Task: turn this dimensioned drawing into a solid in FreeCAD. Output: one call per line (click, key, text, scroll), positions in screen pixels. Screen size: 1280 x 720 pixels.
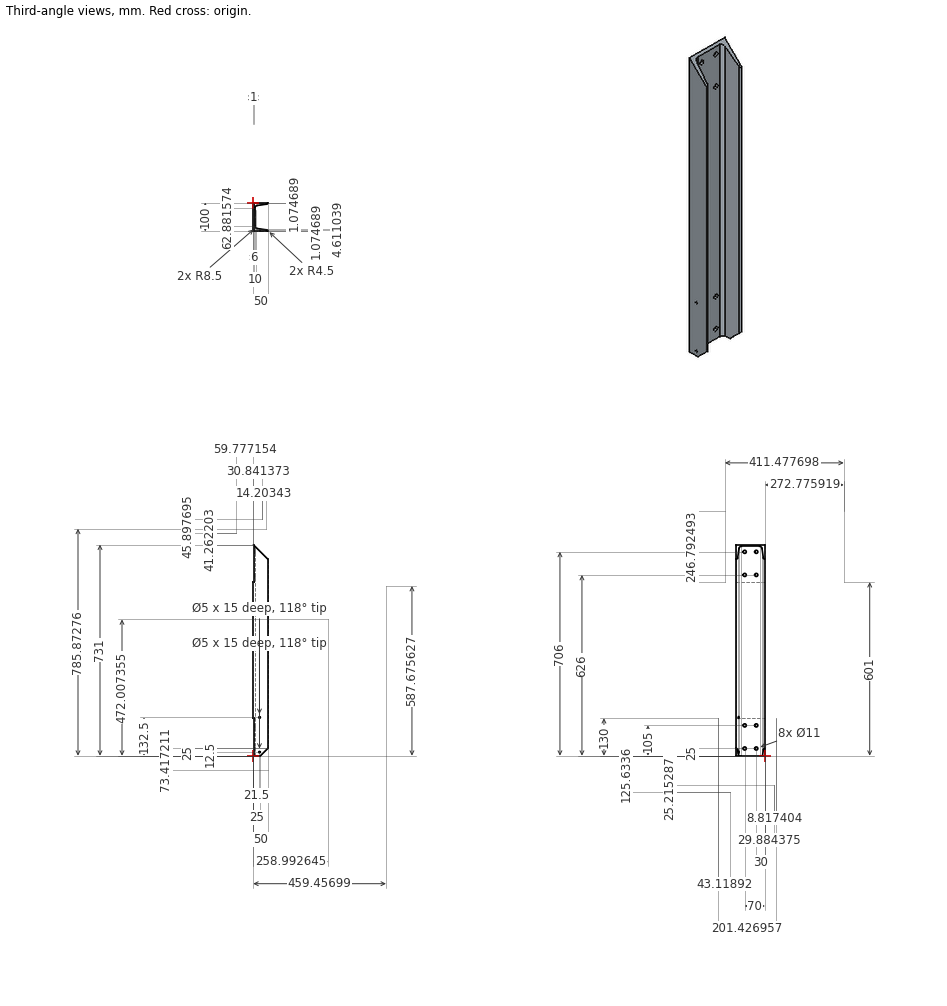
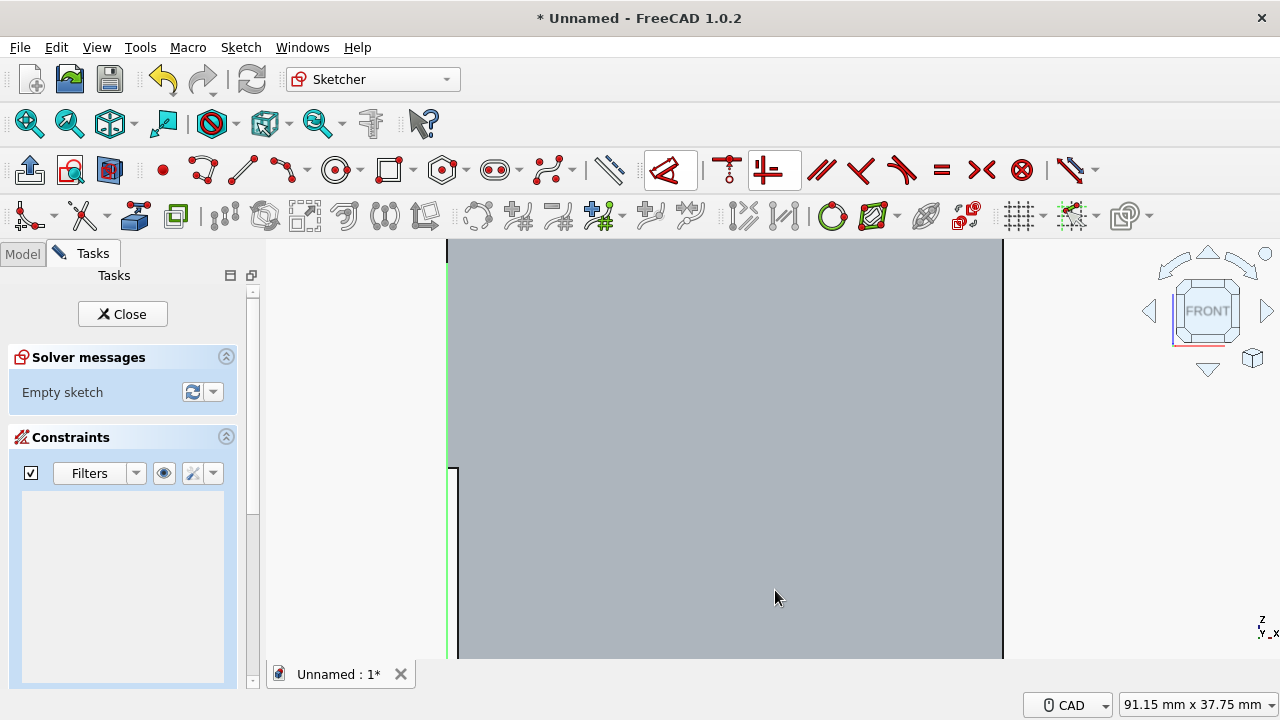
scroll(682, 437, up, 8)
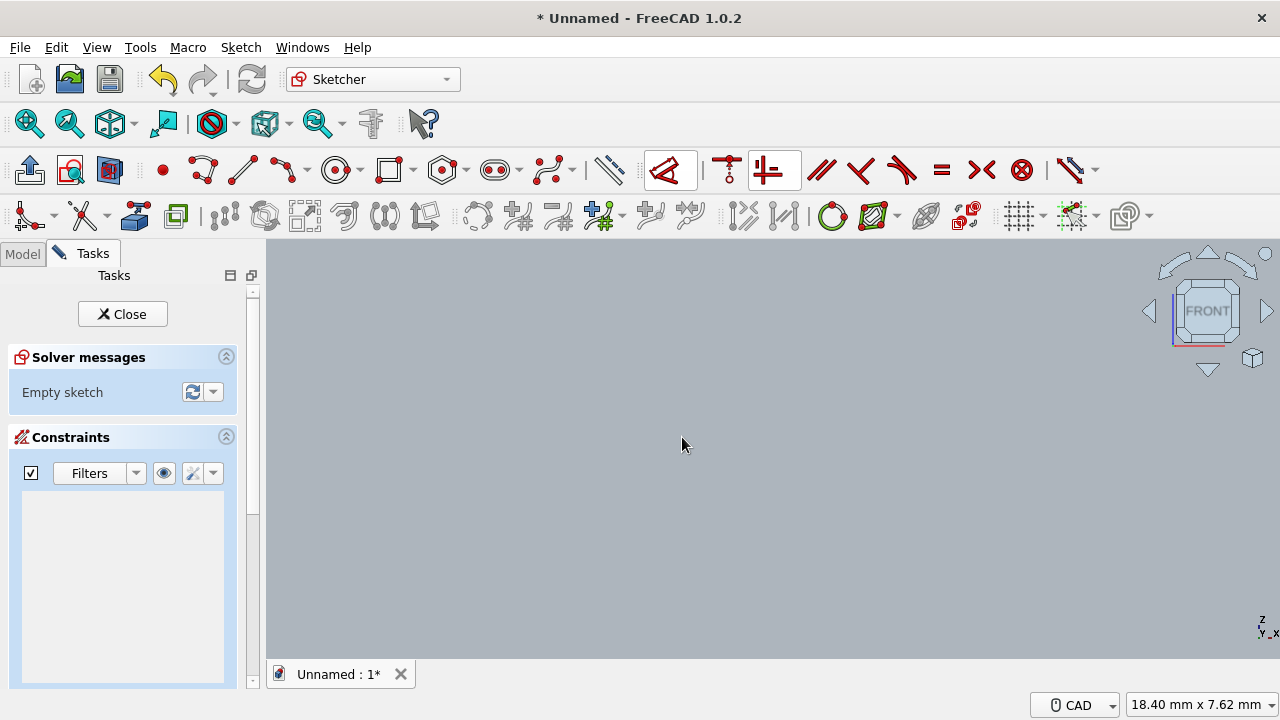
click(336, 170)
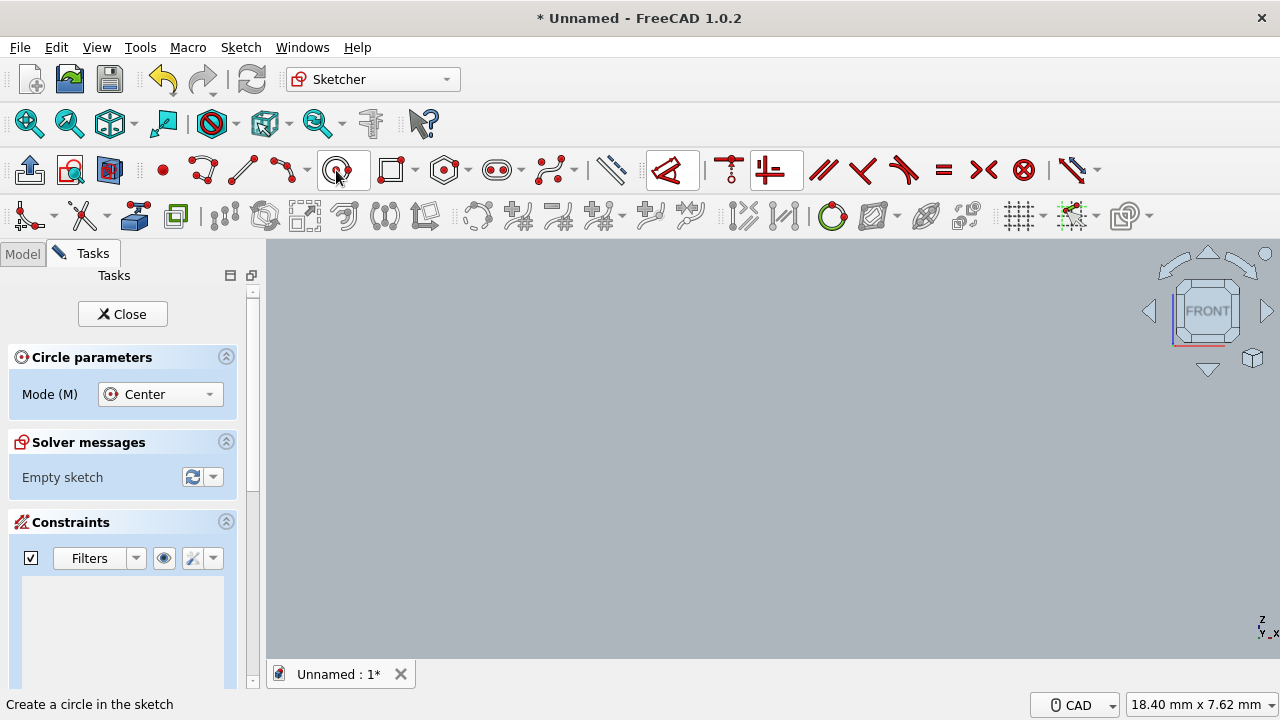
click(702, 449)
move(799, 351)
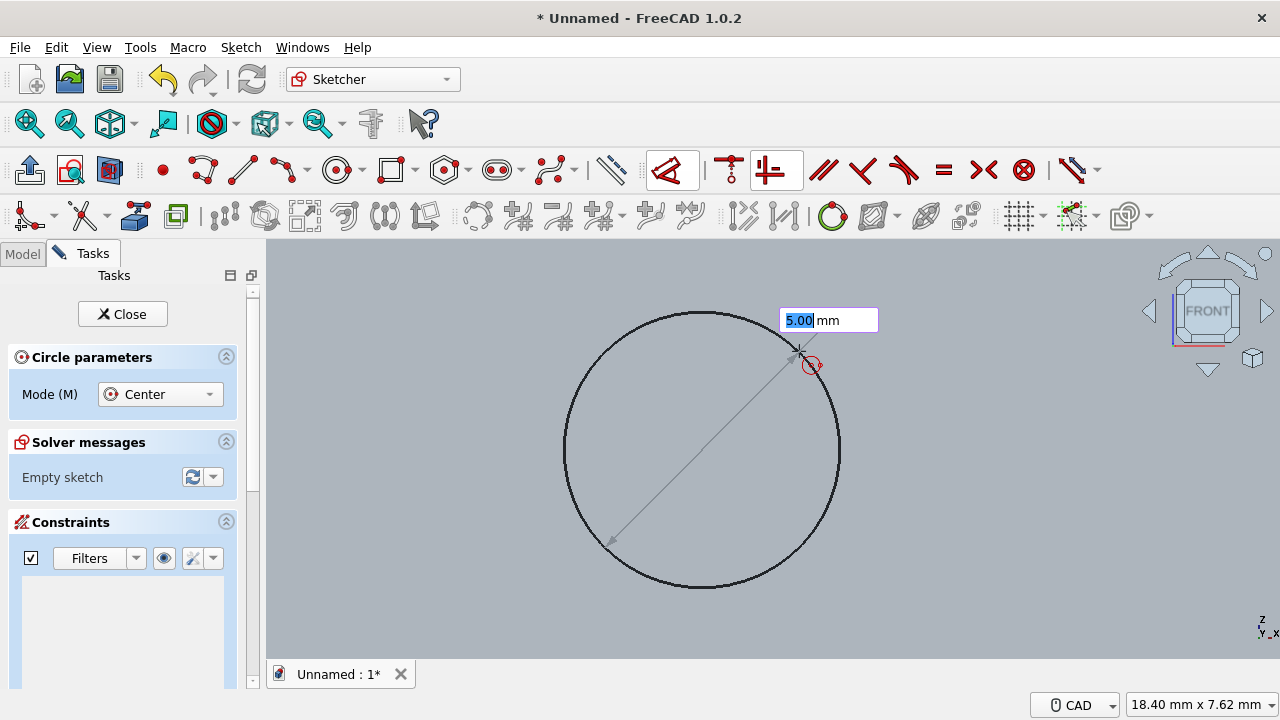
text(5)
key(Return)
key(Escape)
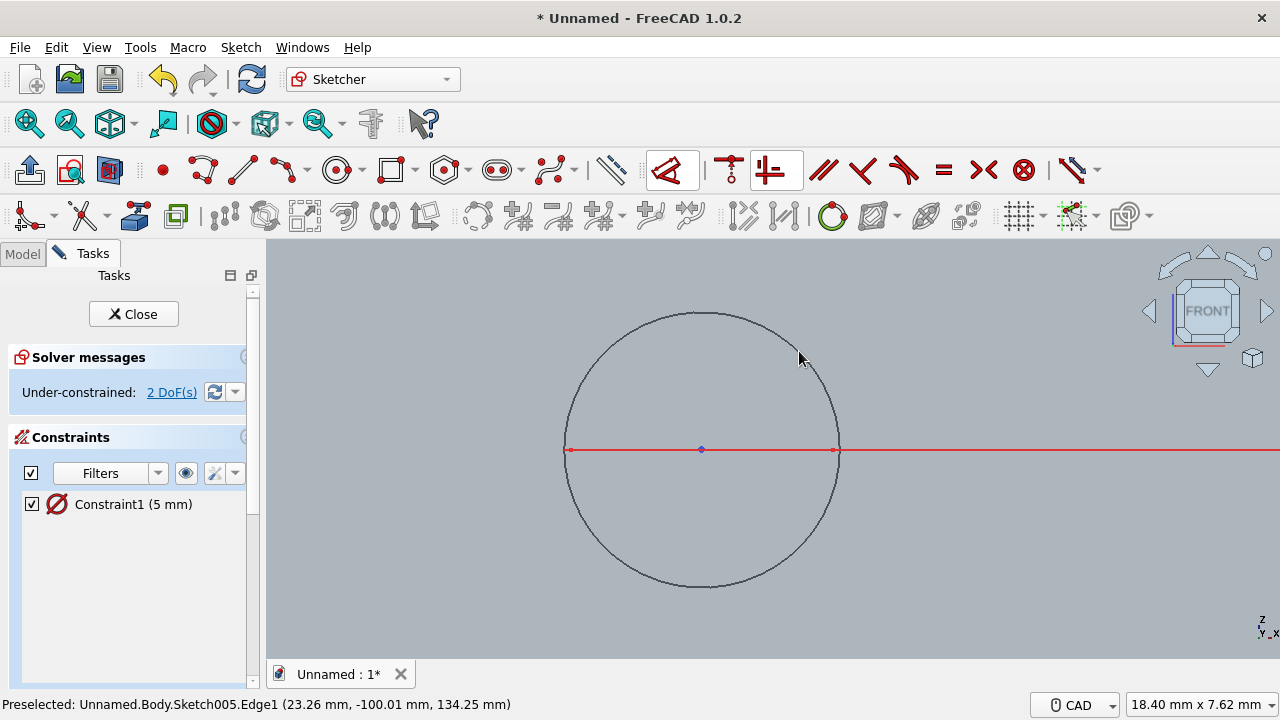
click(702, 450)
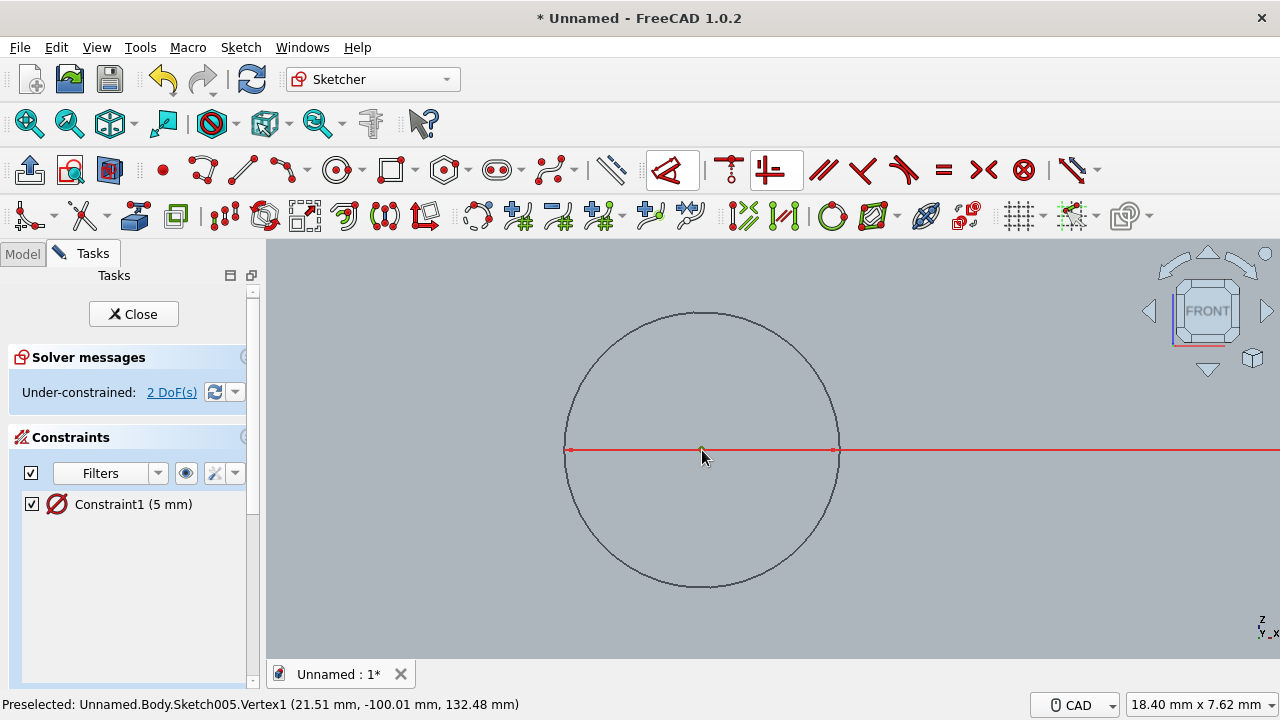
click(694, 170)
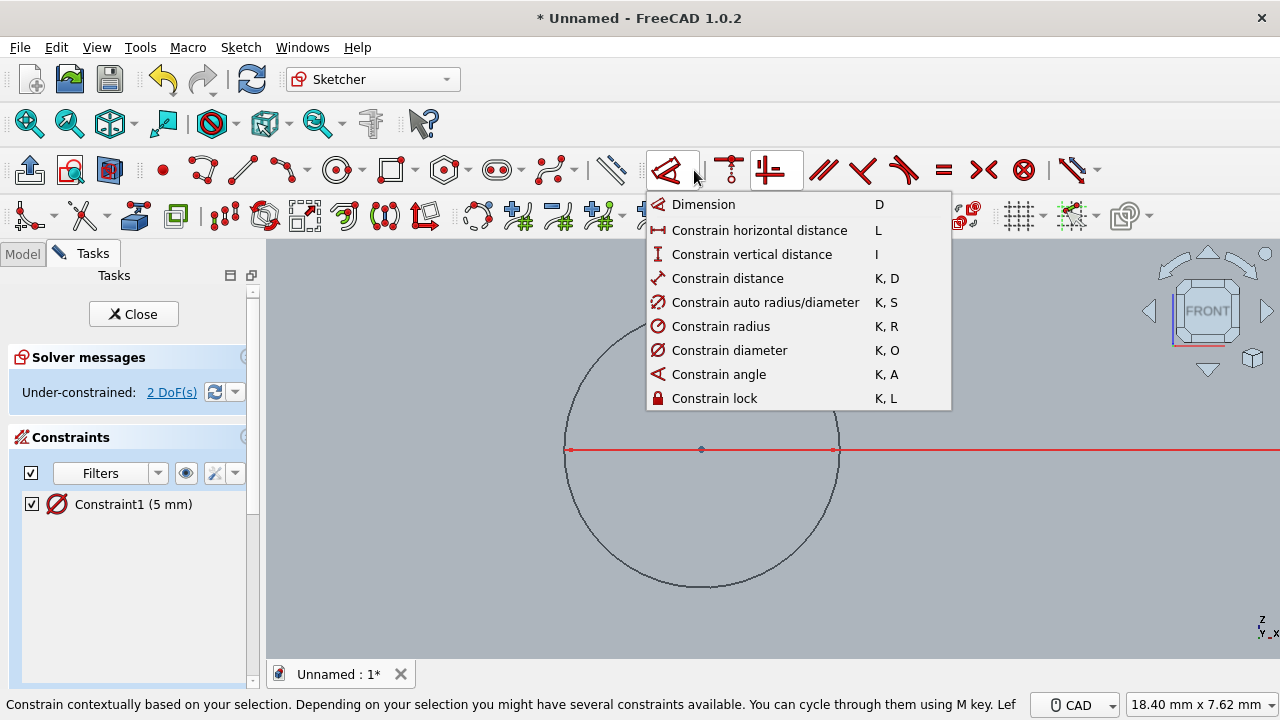
click(799, 230)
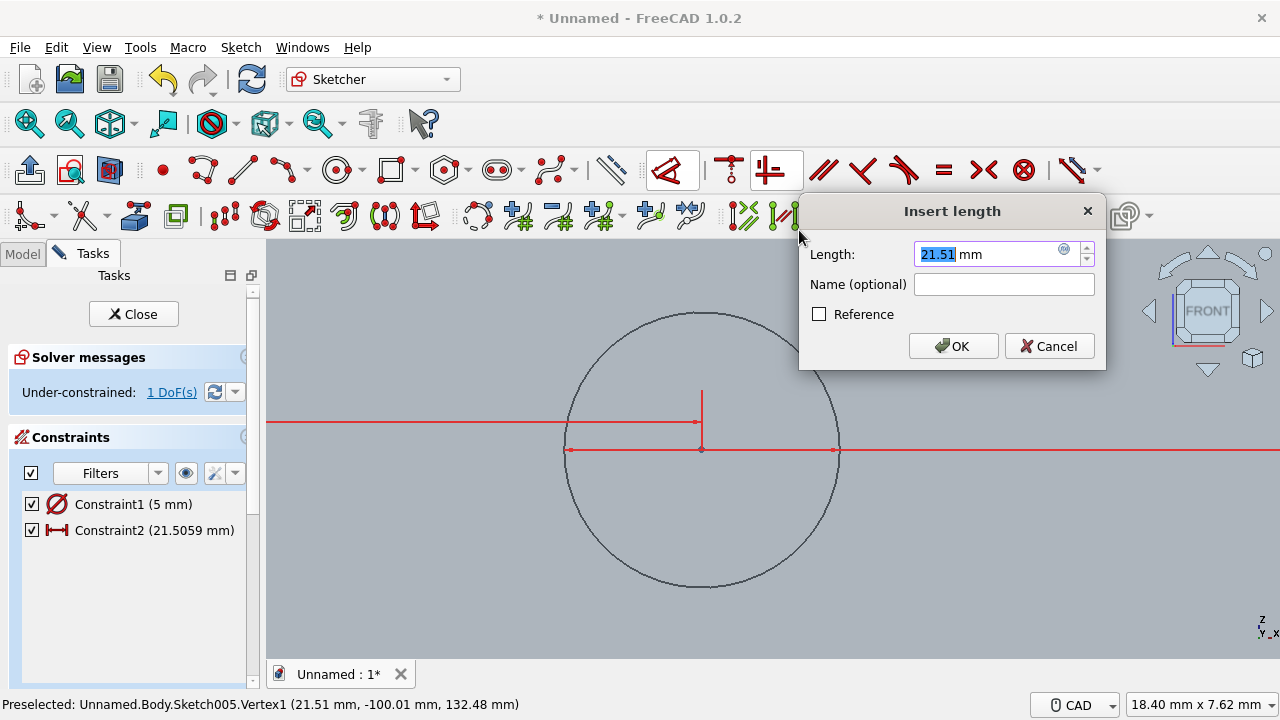
text(21.5)
key(Return)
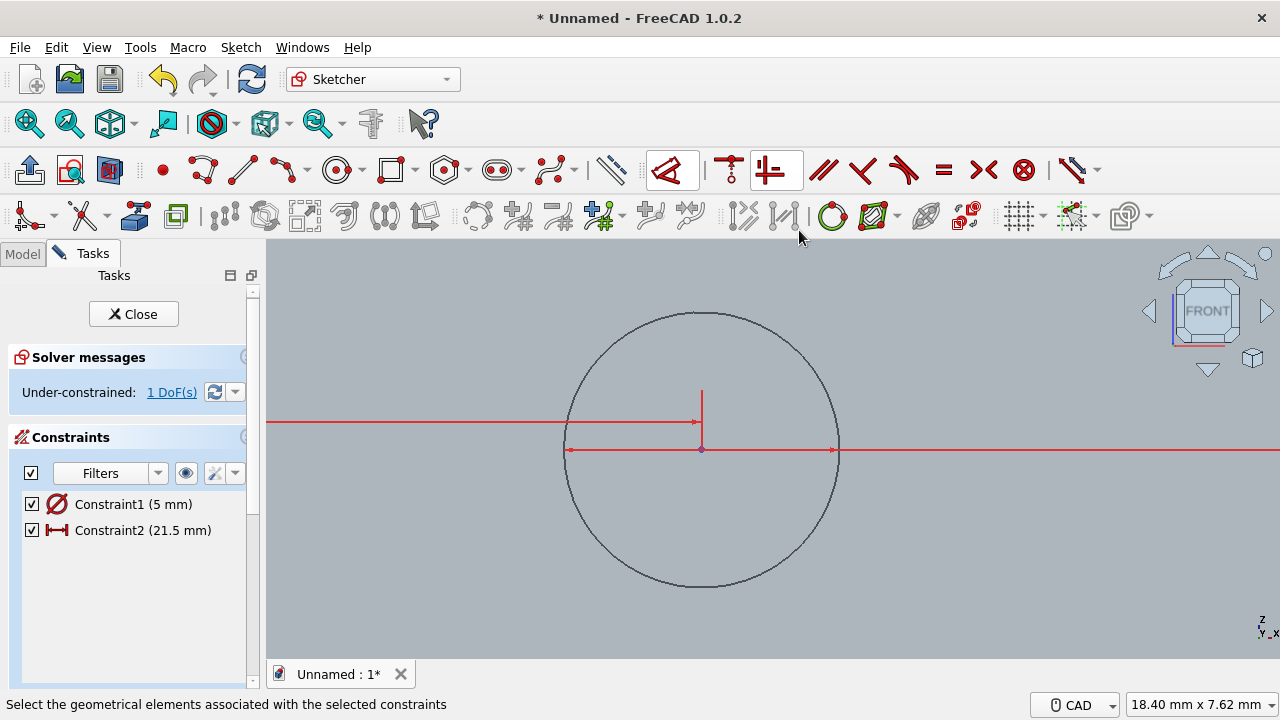
click(702, 450)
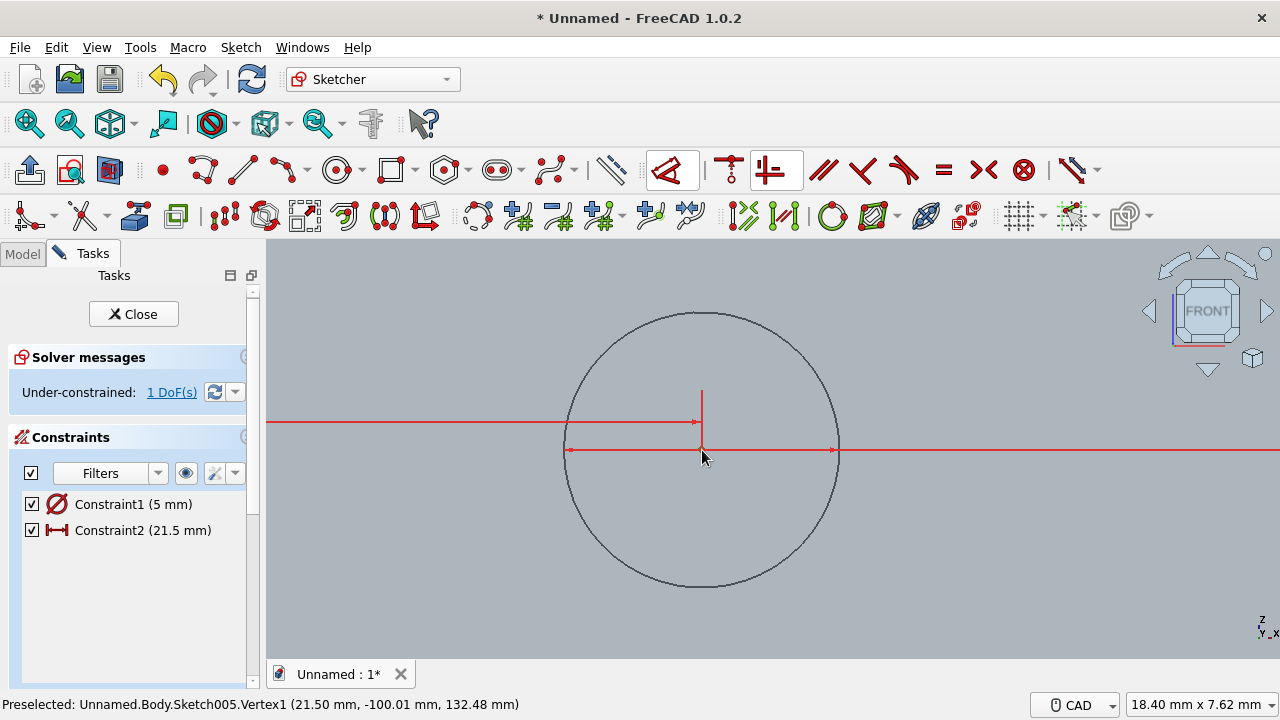
click(694, 170)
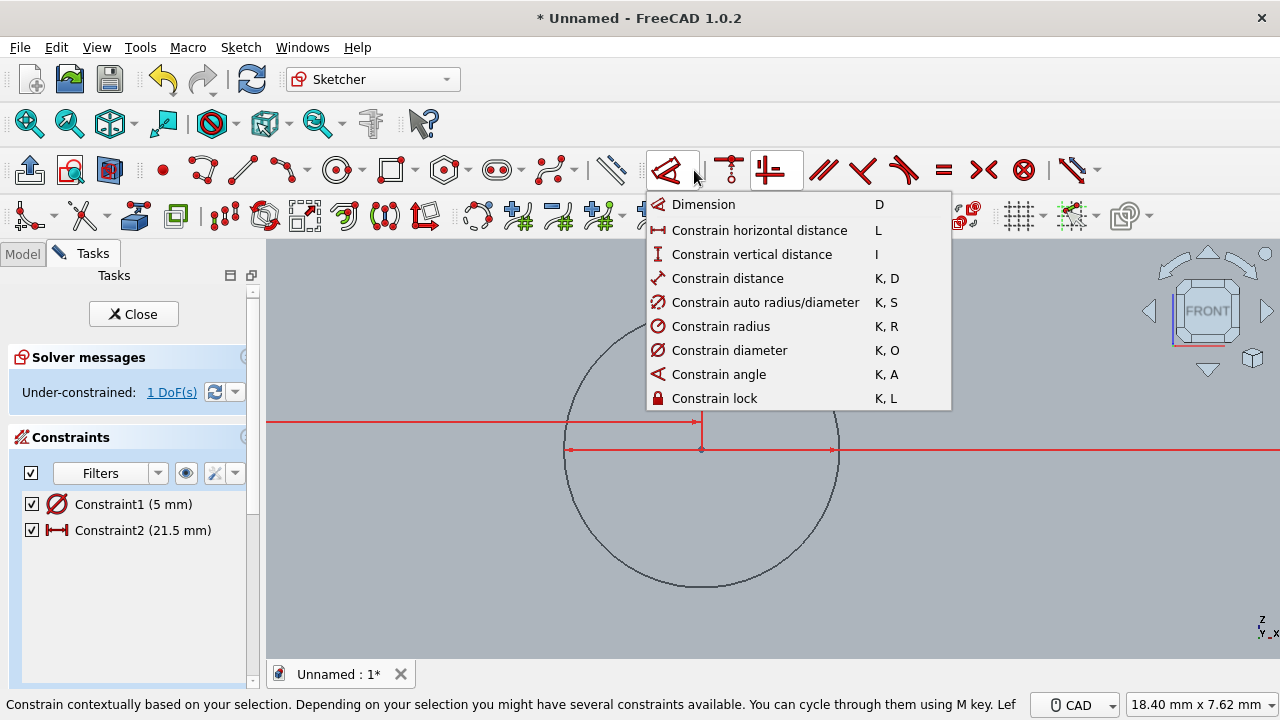
click(799, 254)